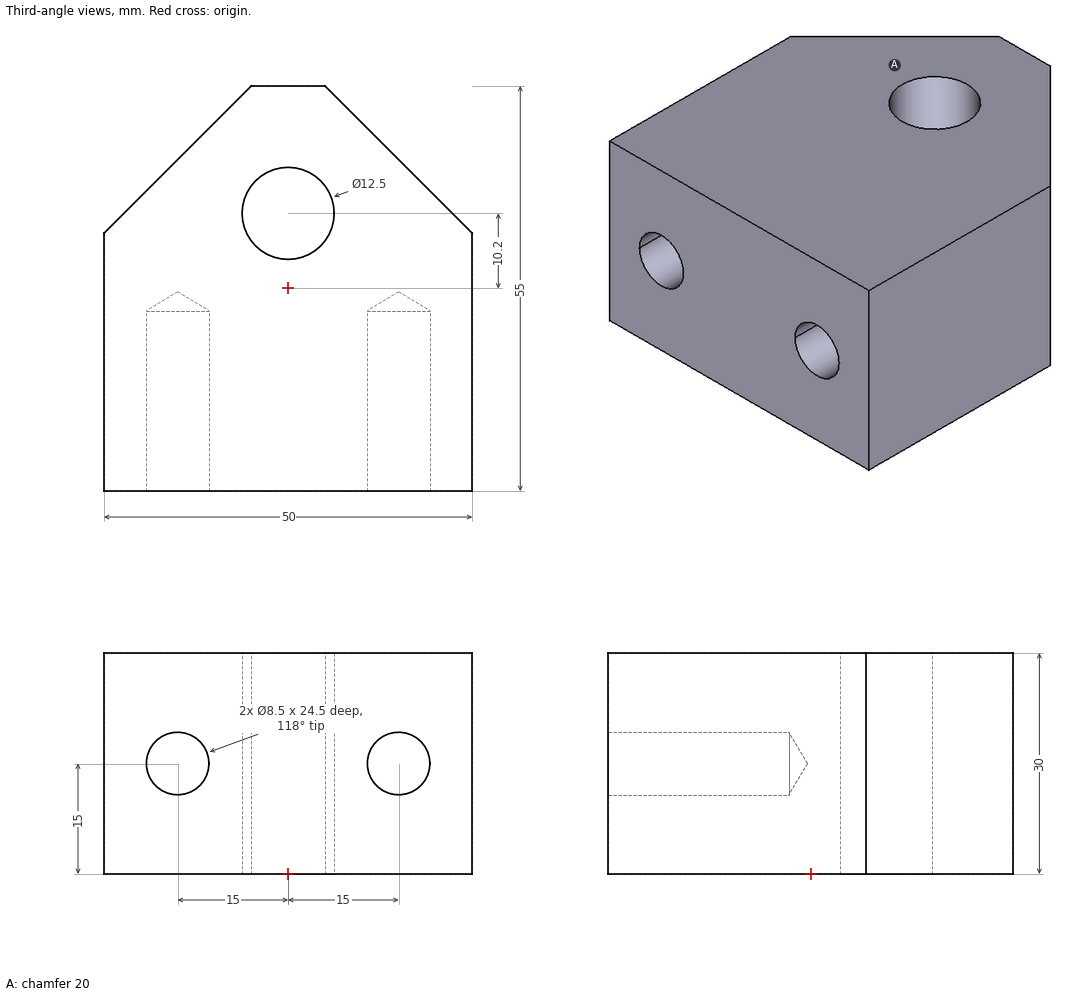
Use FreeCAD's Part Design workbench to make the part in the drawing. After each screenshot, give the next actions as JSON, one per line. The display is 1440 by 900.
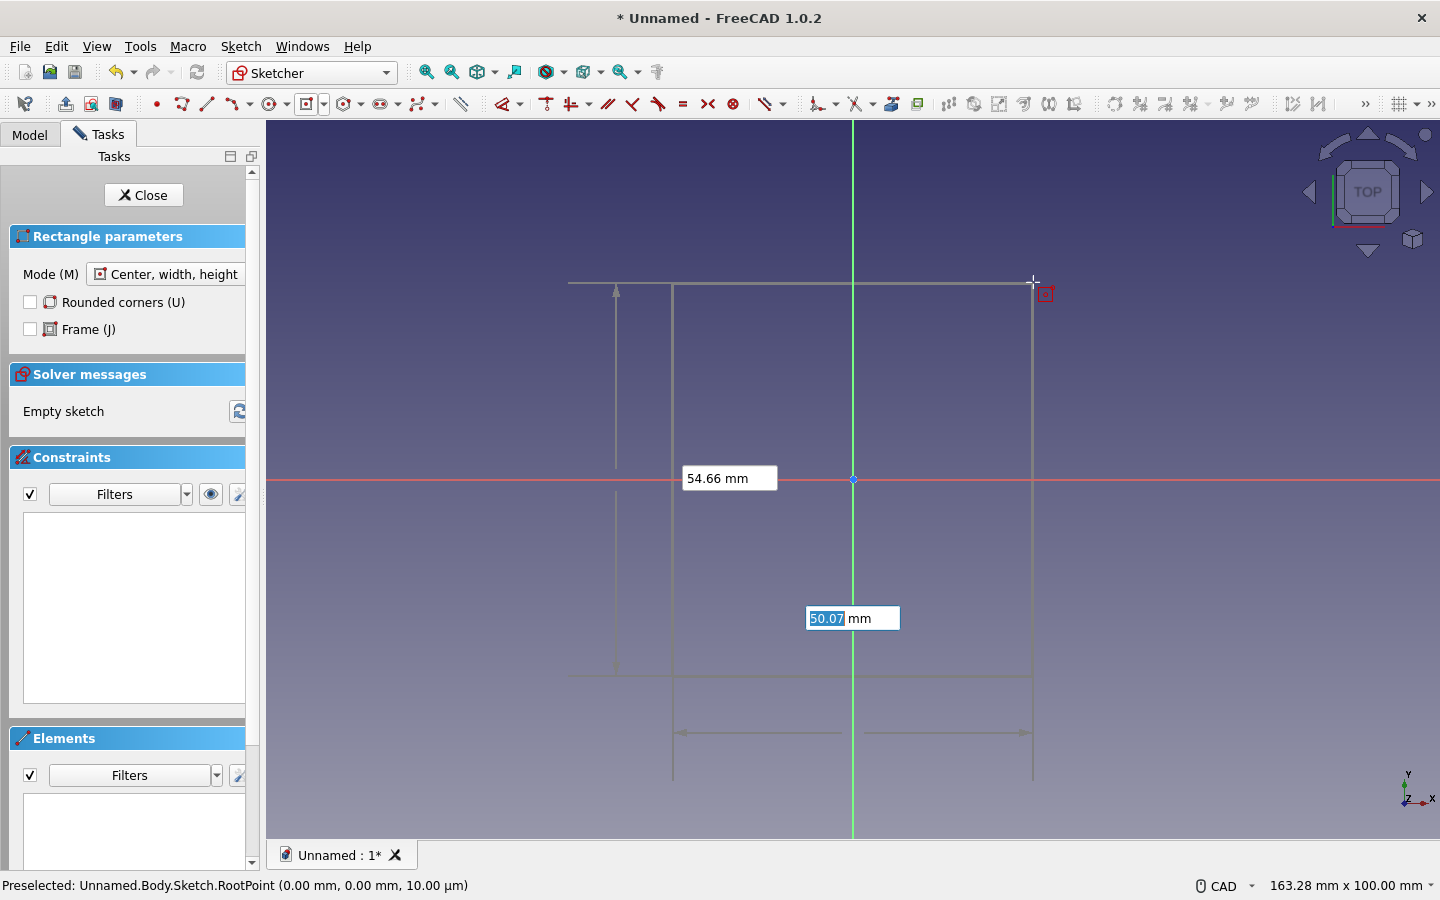
{"action": "type", "text": "50"}
{"action": "key", "text": "Tab"}
{"action": "type", "text": "55"}
{"action": "key", "text": "Return"}
{"action": "key", "text": "Escape"}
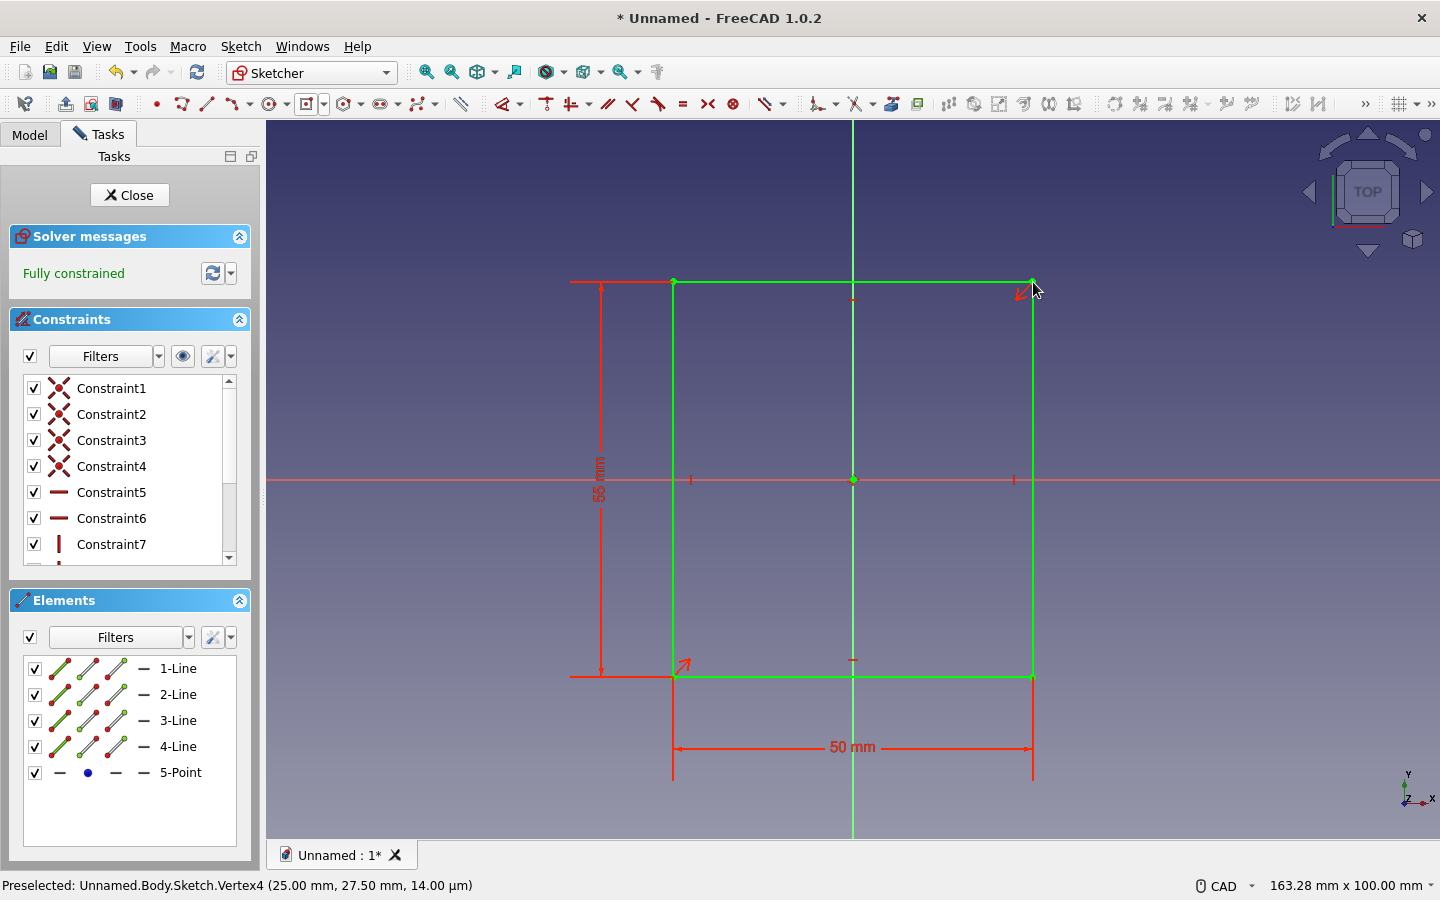
{"action": "left_click", "coordinate": [130, 195]}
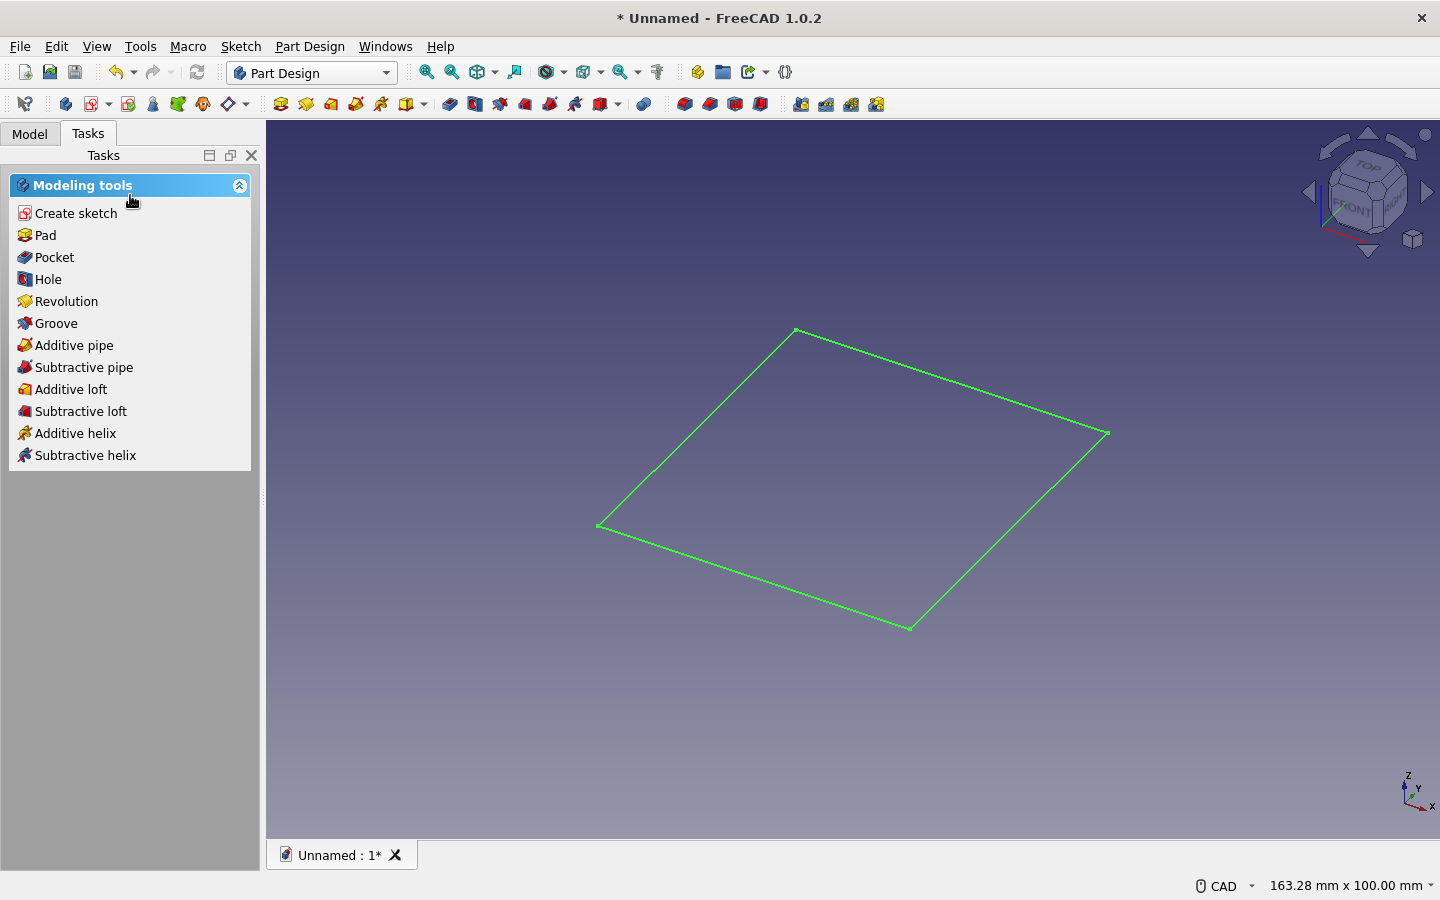
{"action": "left_click", "coordinate": [281, 104]}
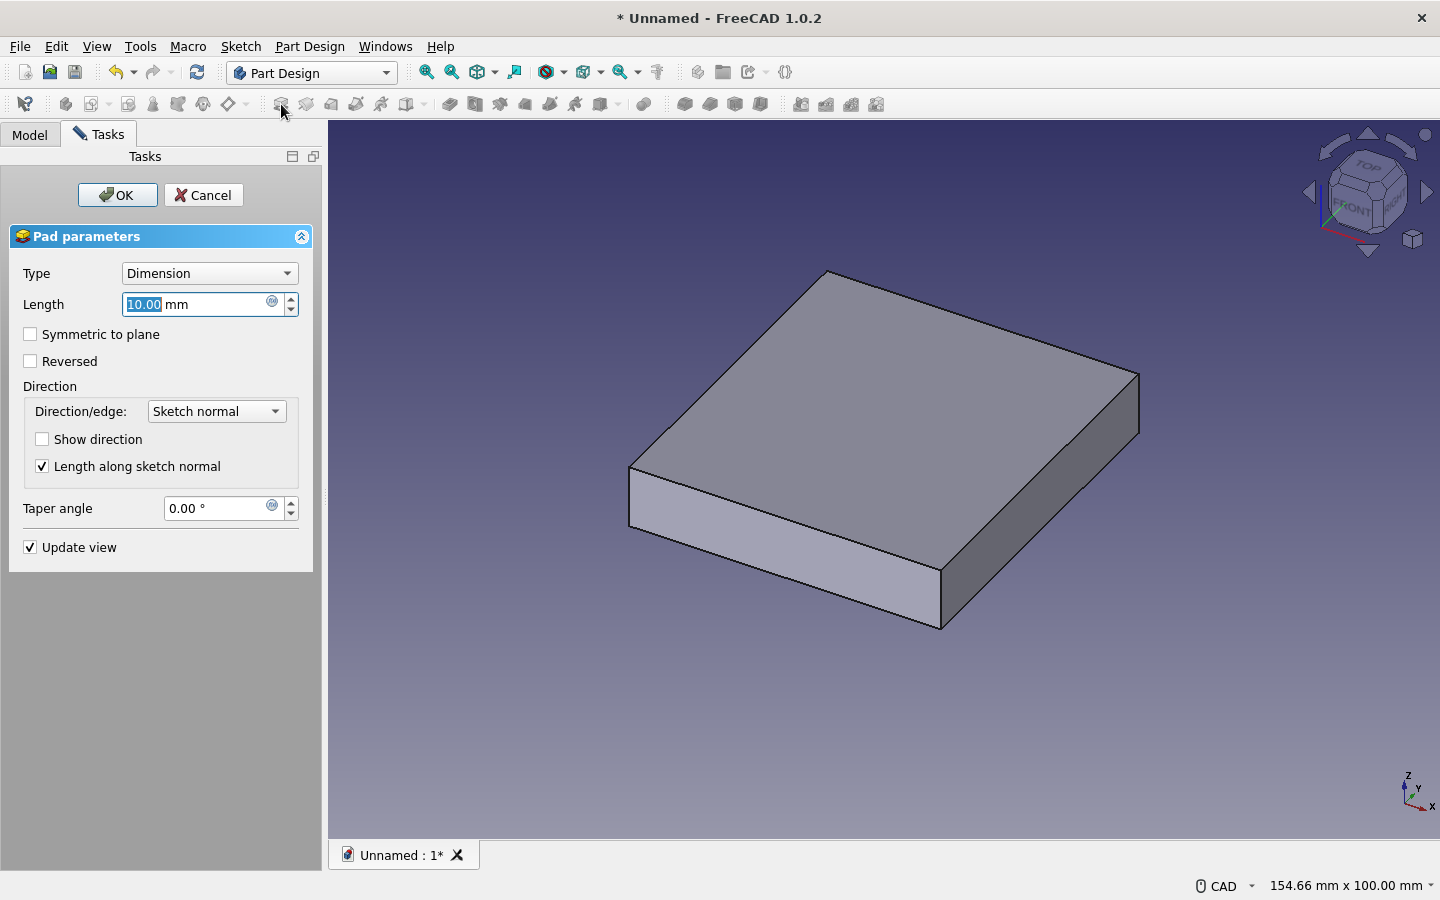
{"action": "type", "text": "30"}
{"action": "key", "text": "Tab"}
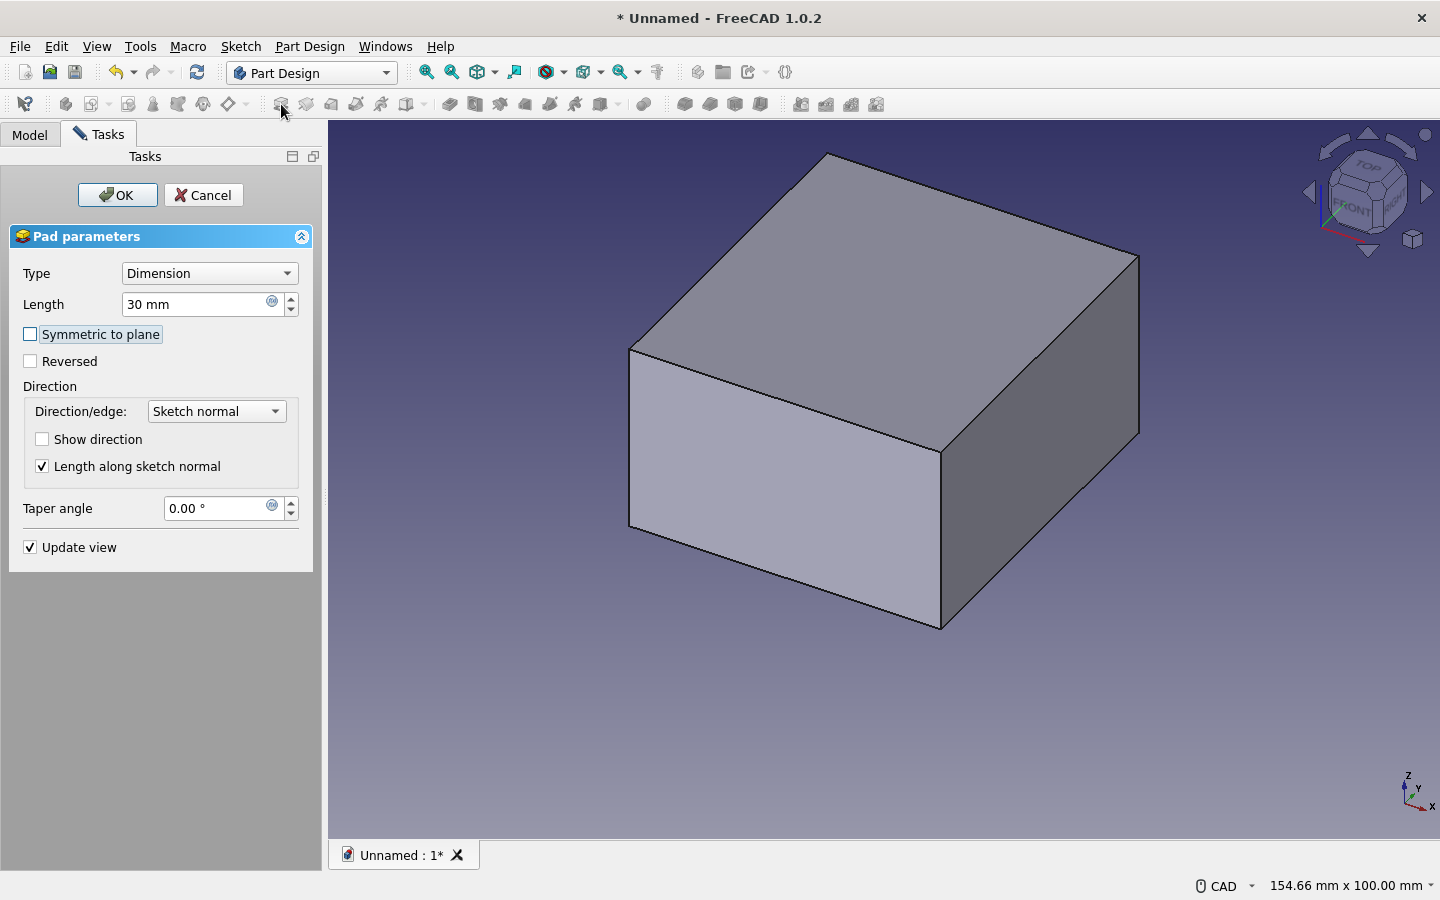
{"action": "left_click", "coordinate": [118, 195]}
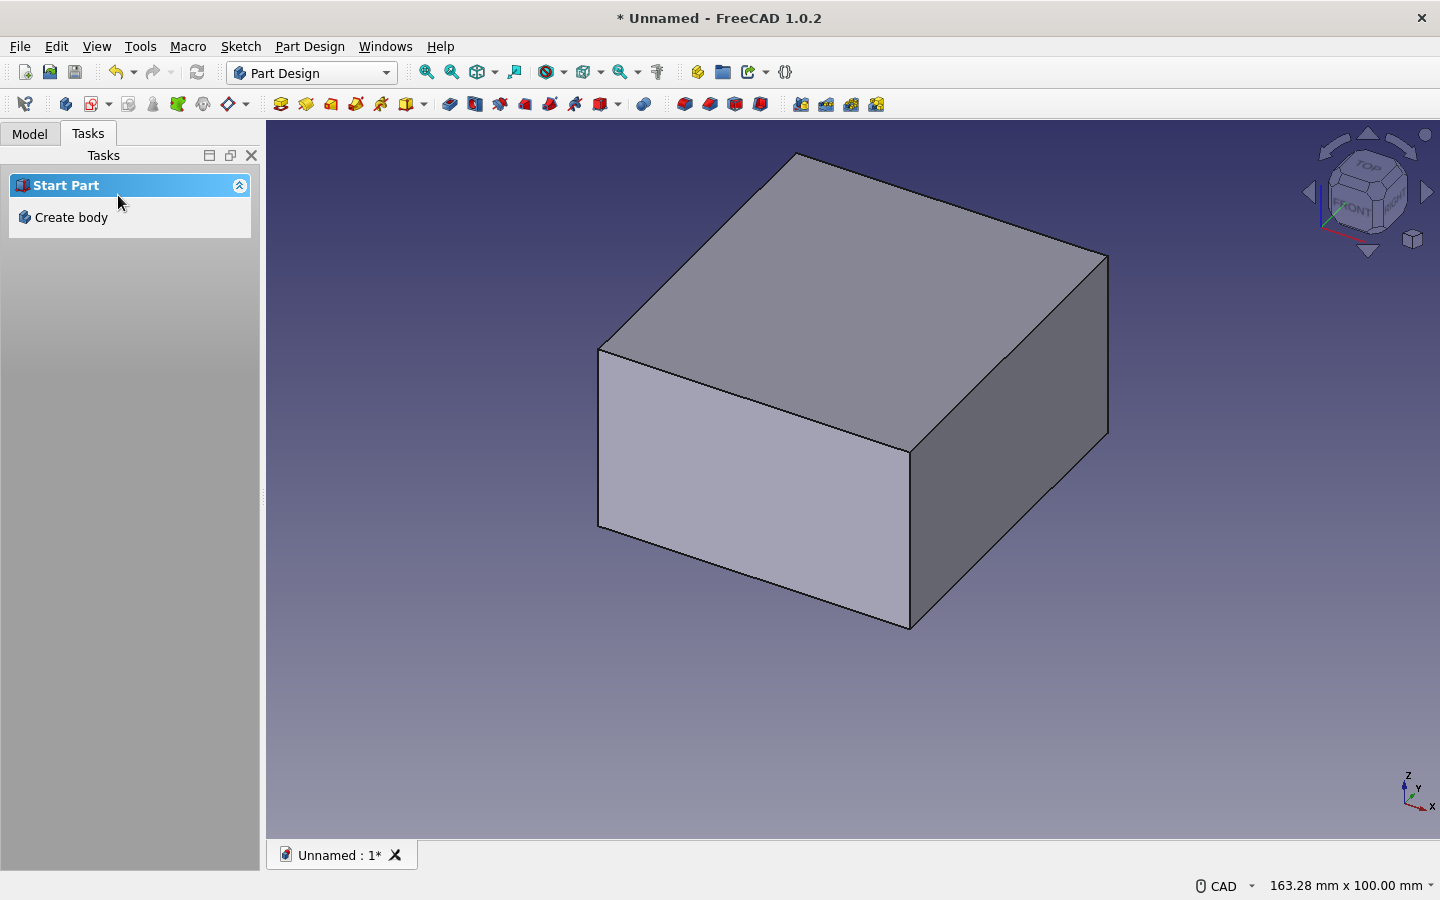
{"action": "key", "text": "0"}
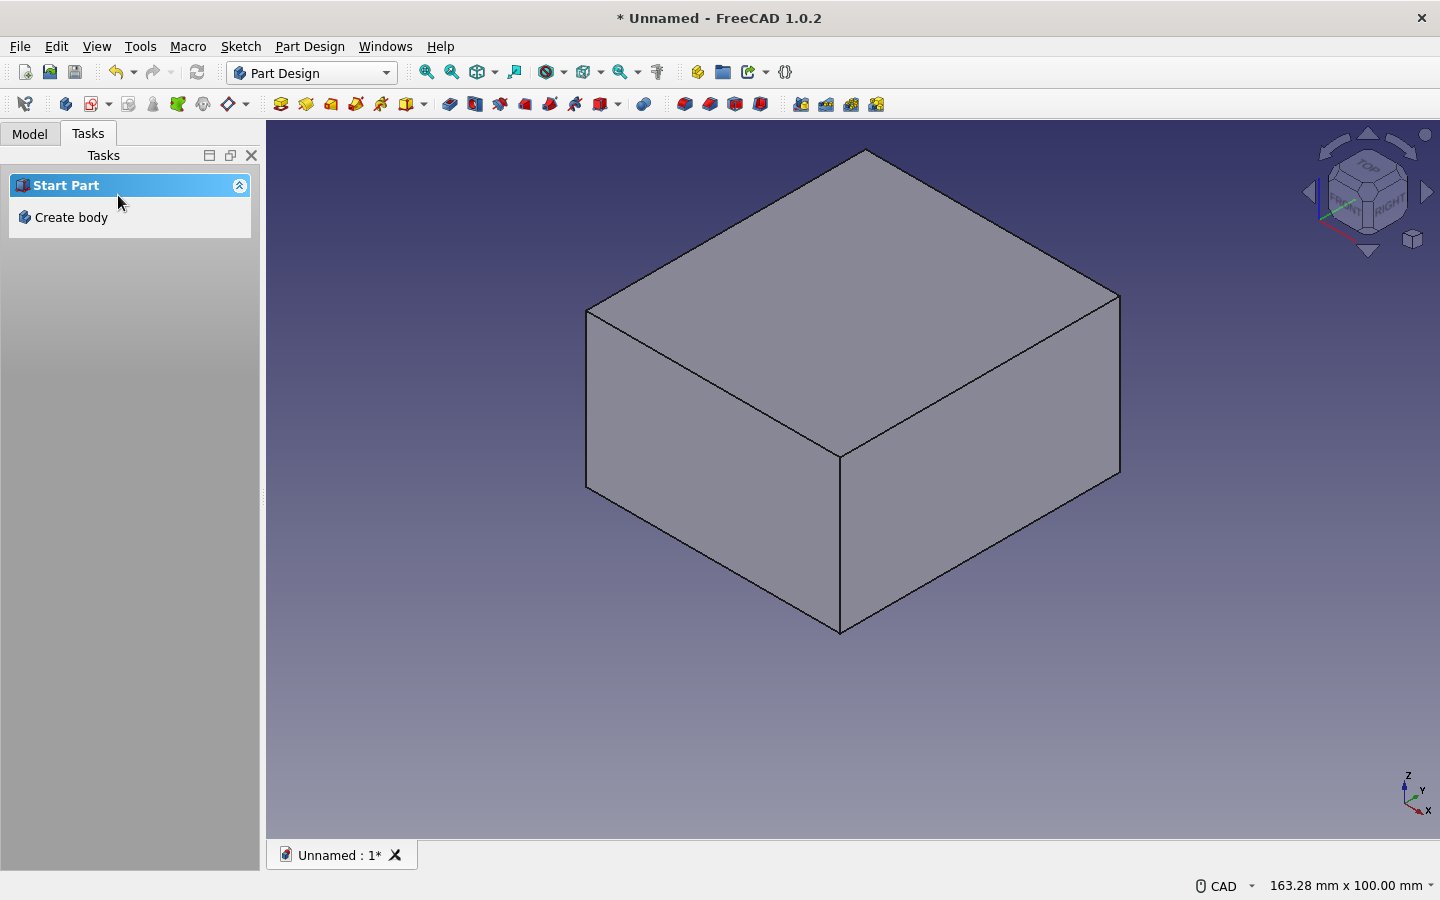
{"action": "key", "text": "2"}